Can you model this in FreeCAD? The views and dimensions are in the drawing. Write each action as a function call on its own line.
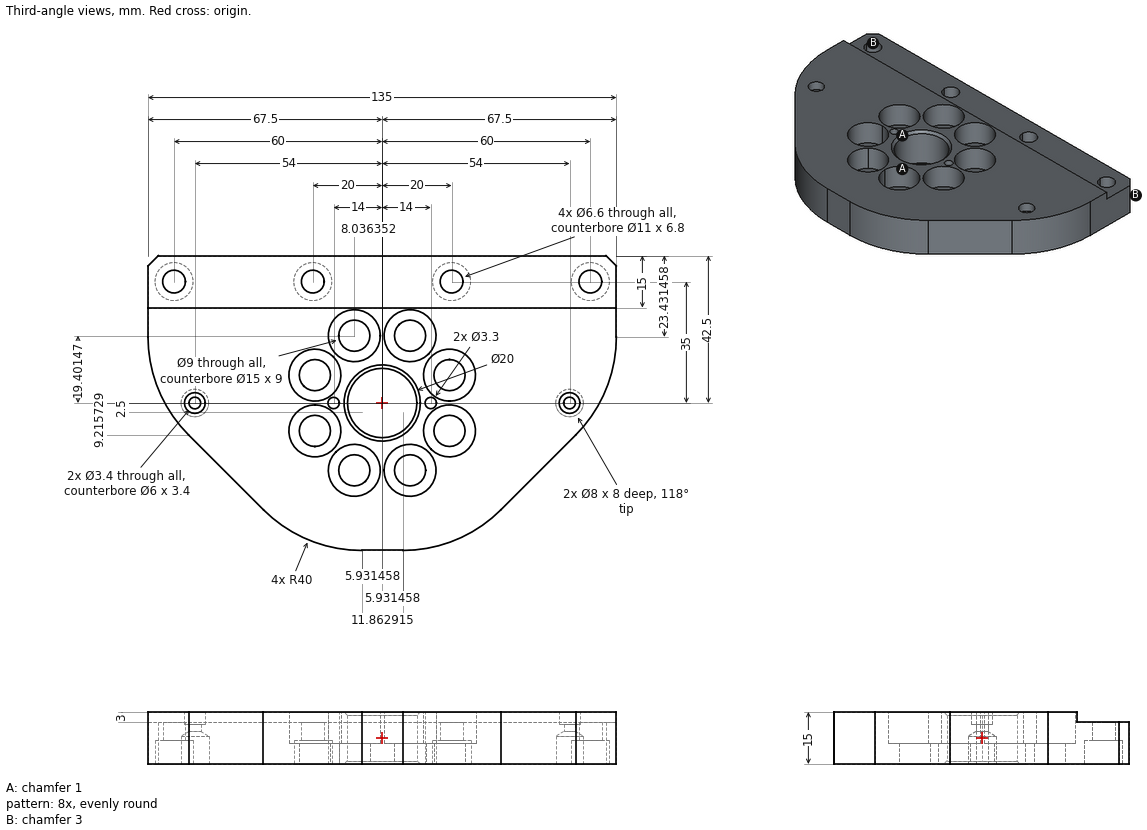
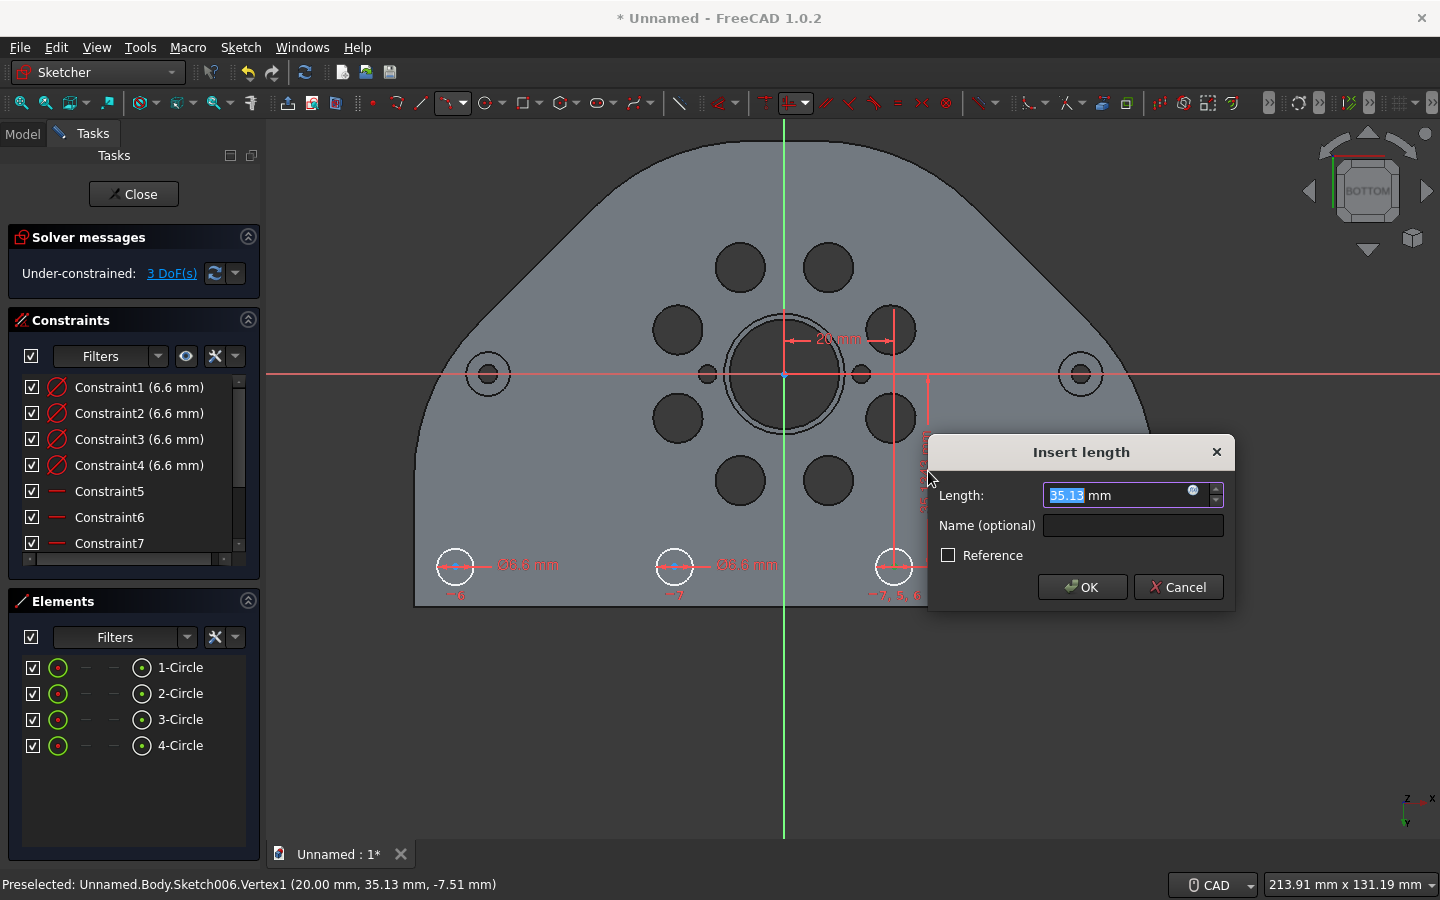
text(35)
key(Return)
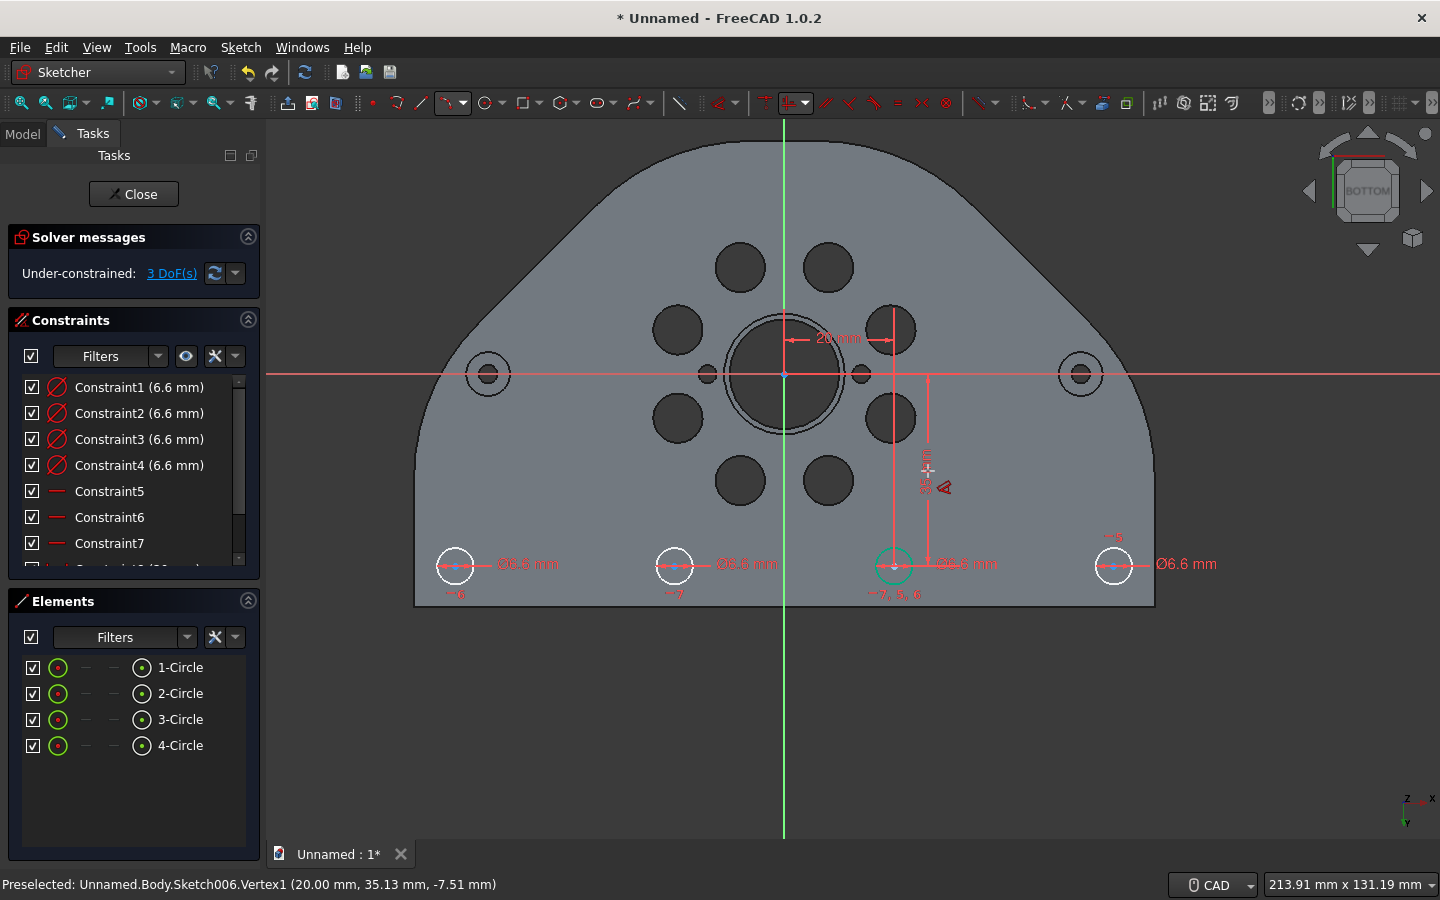
click(1114, 566)
click(949, 340)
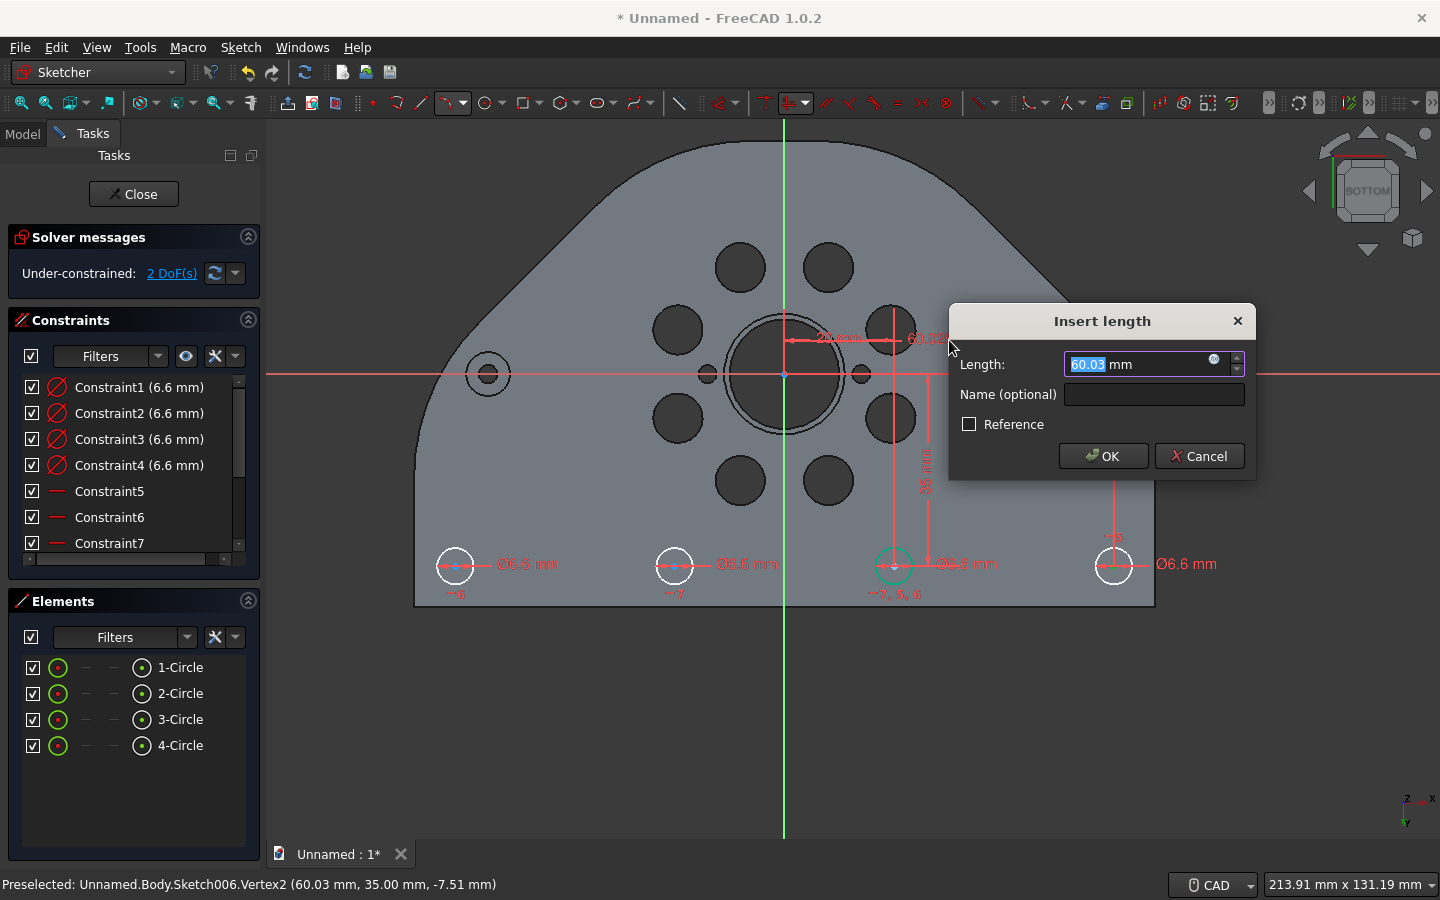
text(60)
key(Return)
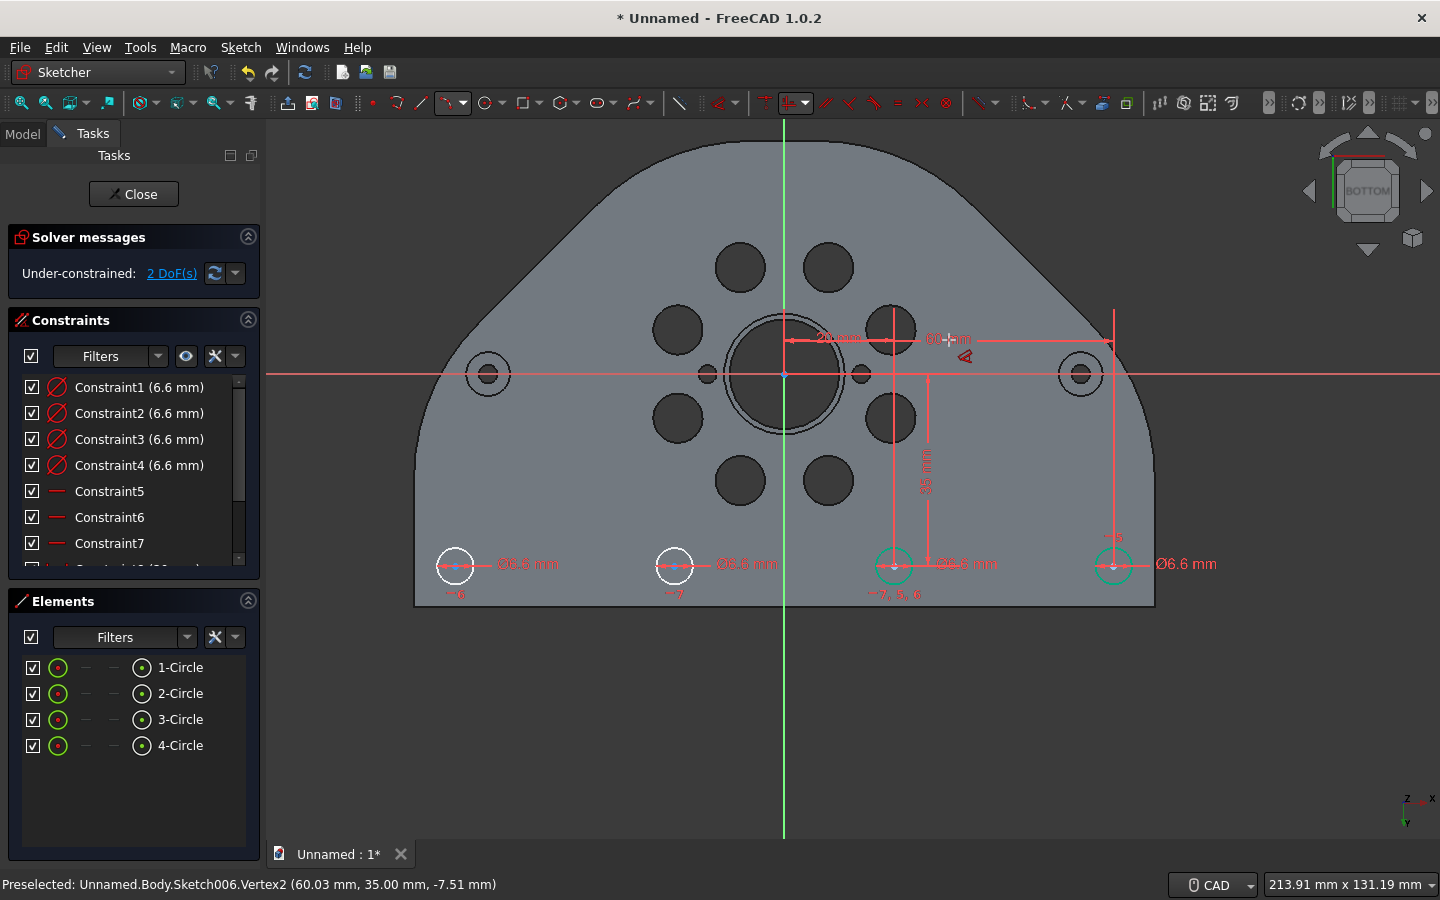
click(455, 566)
click(620, 340)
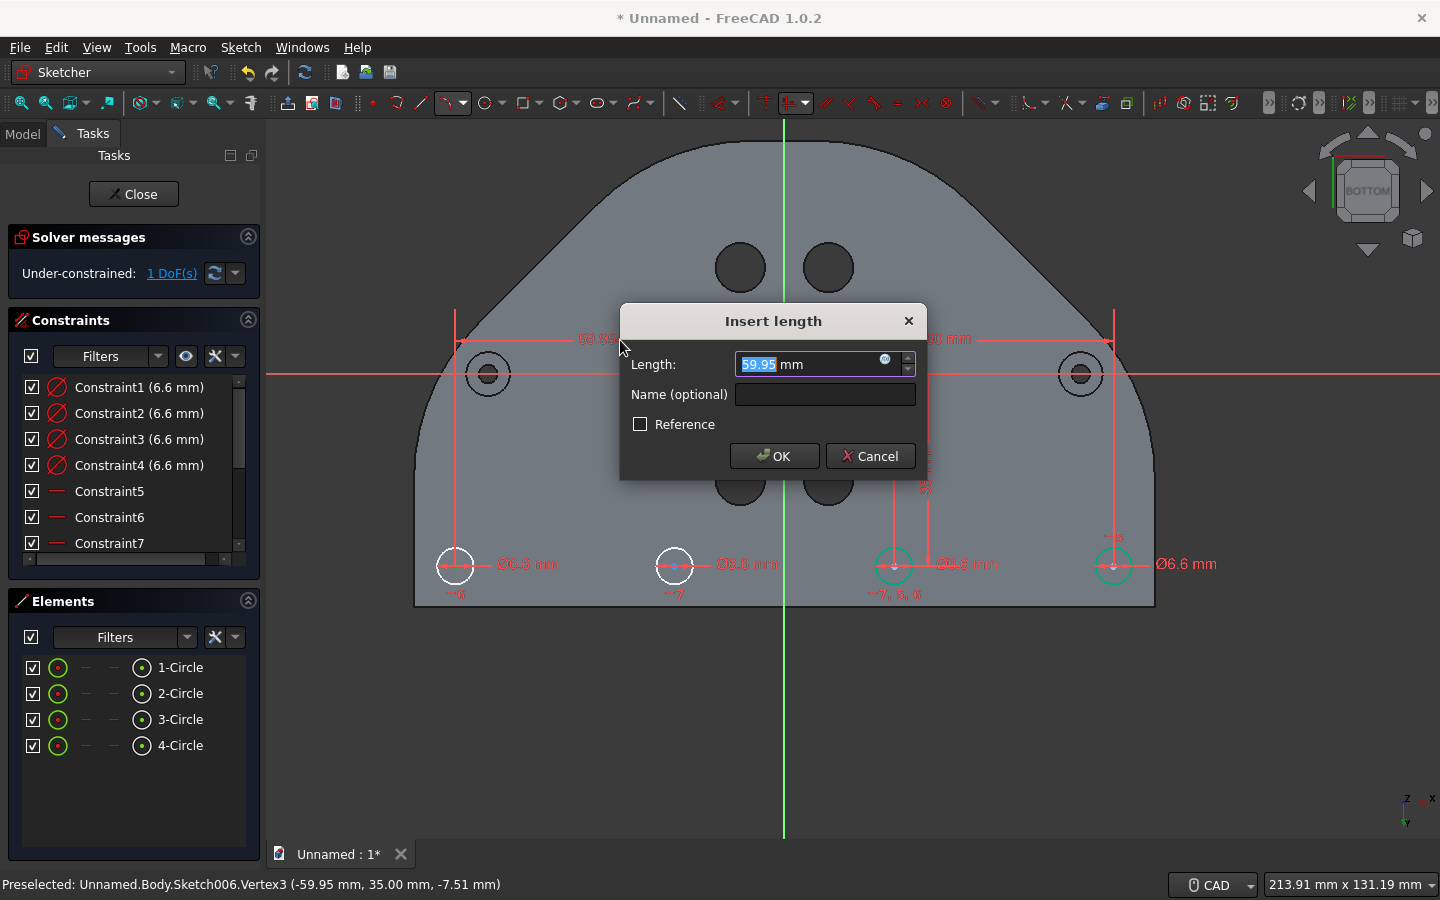
text(60)
key(Return)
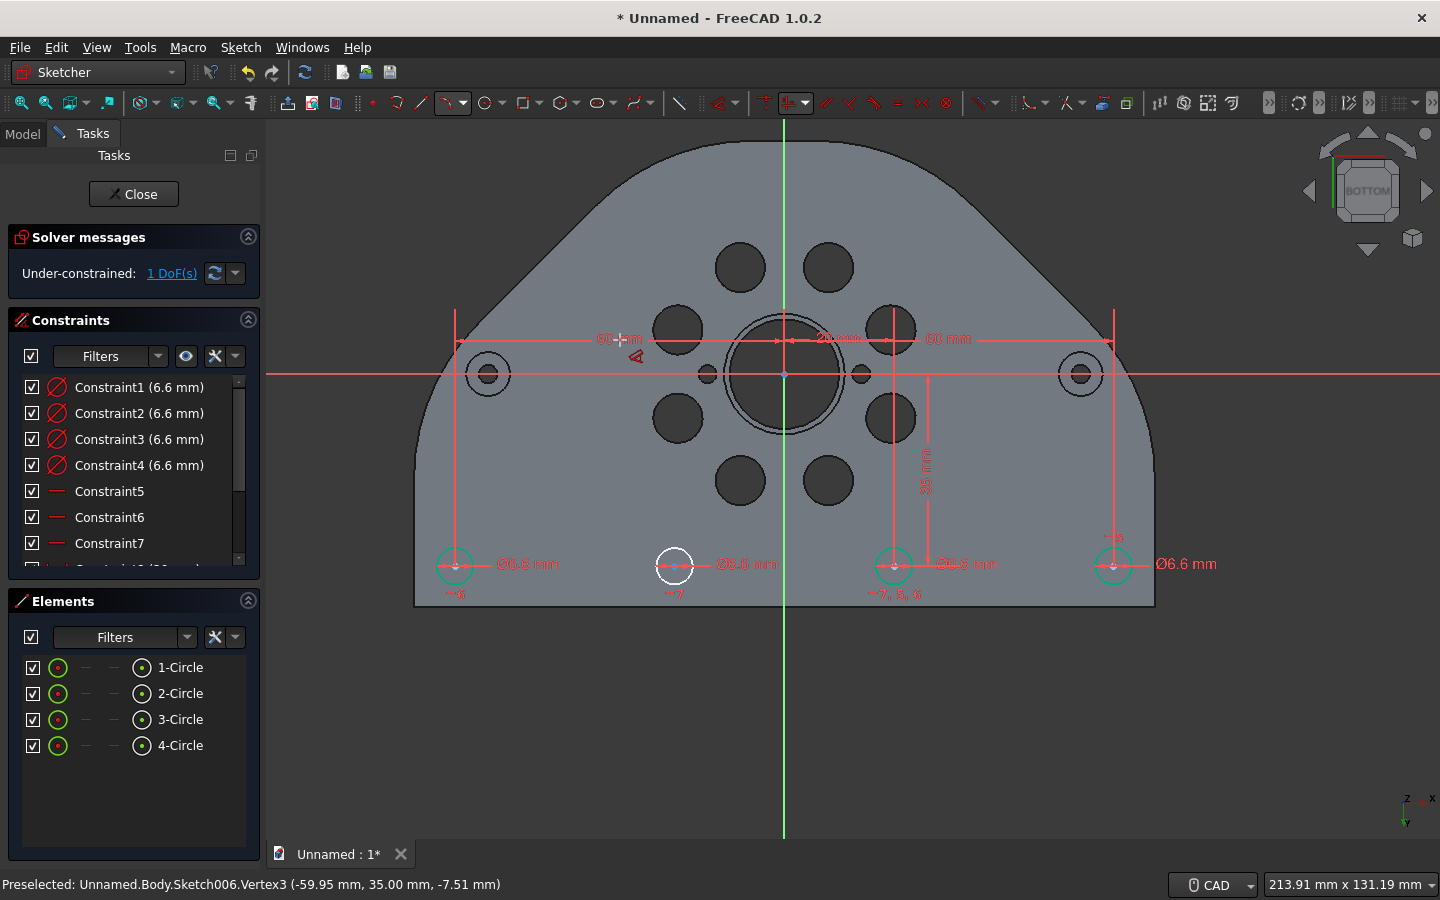
click(675, 566)
click(730, 340)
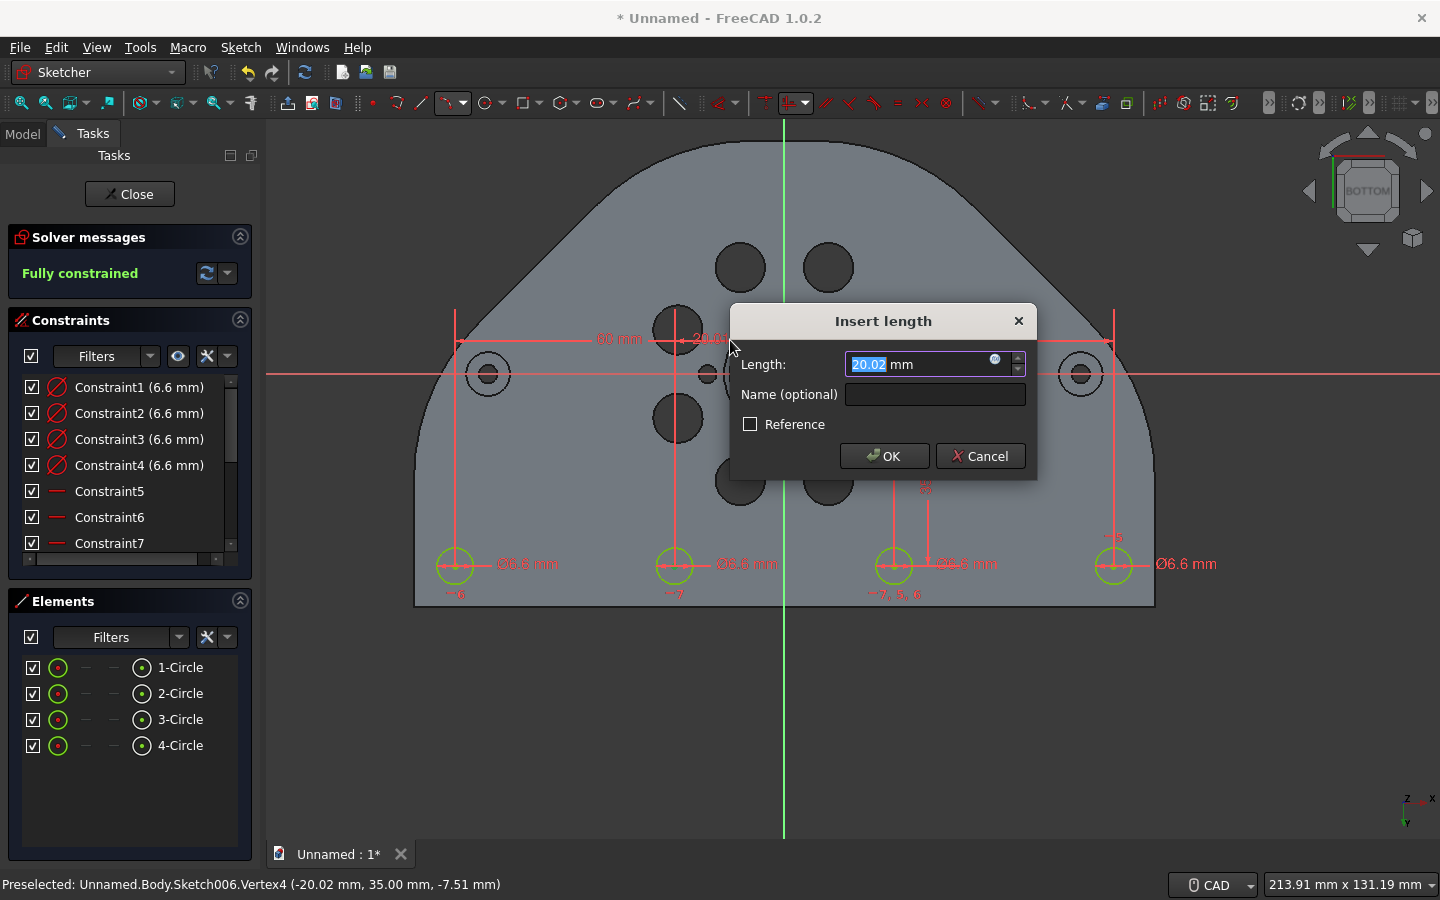
text(20)
key(Return)
key(Escape)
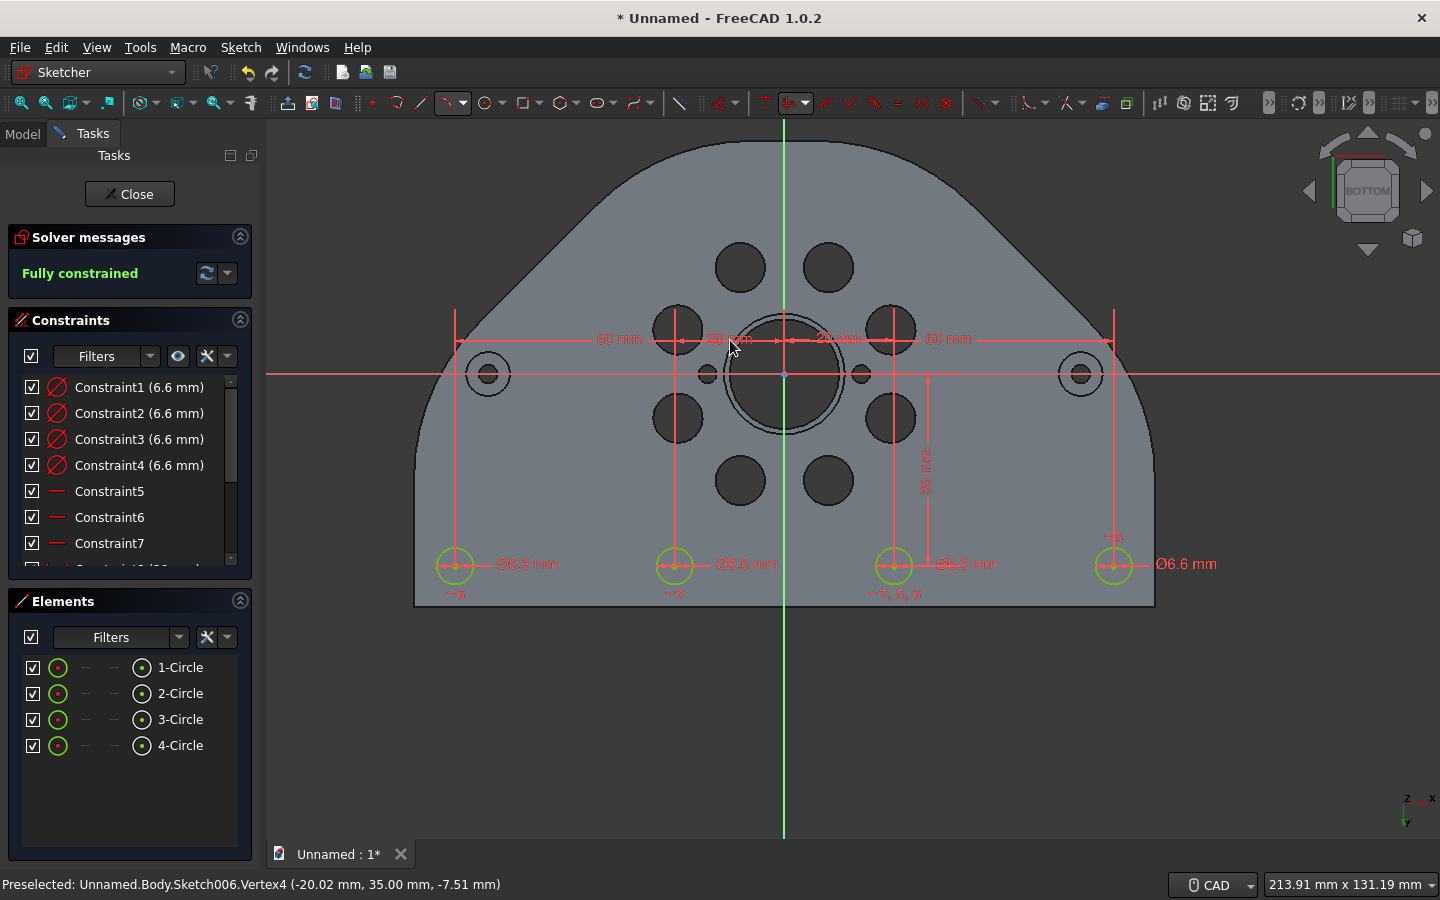
click(130, 194)